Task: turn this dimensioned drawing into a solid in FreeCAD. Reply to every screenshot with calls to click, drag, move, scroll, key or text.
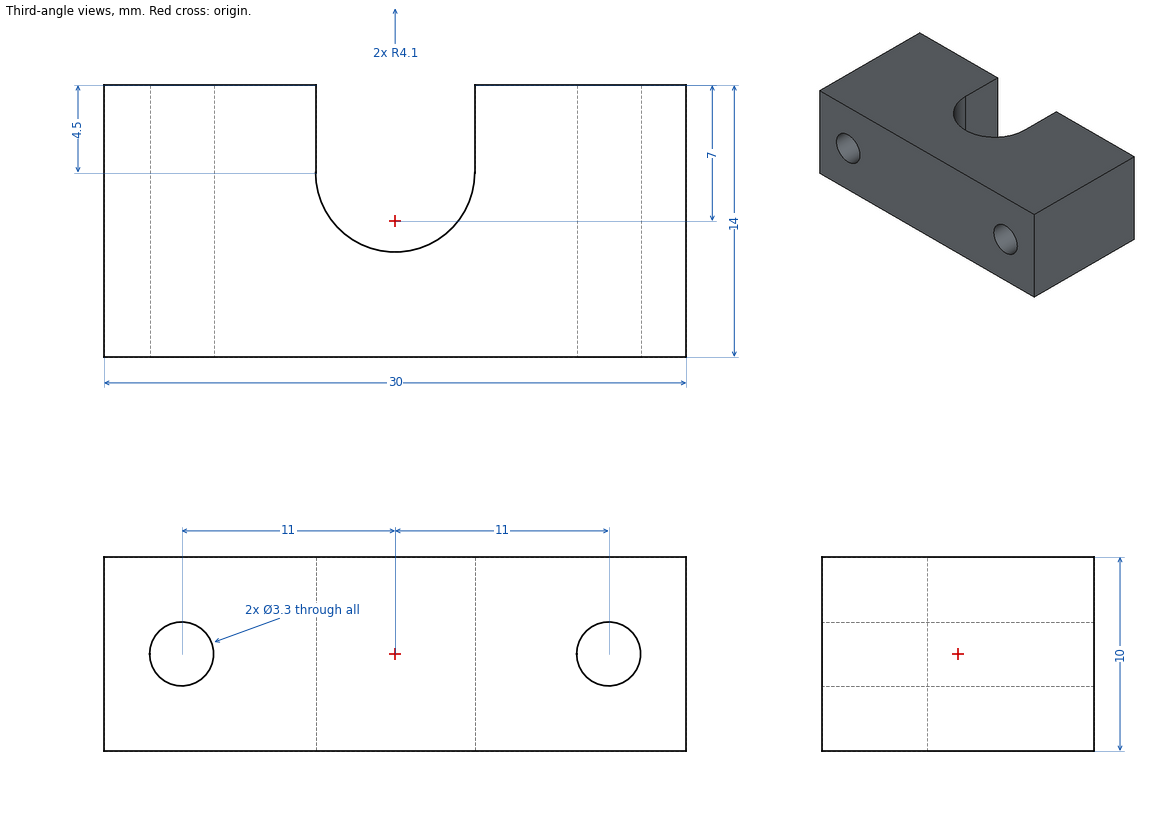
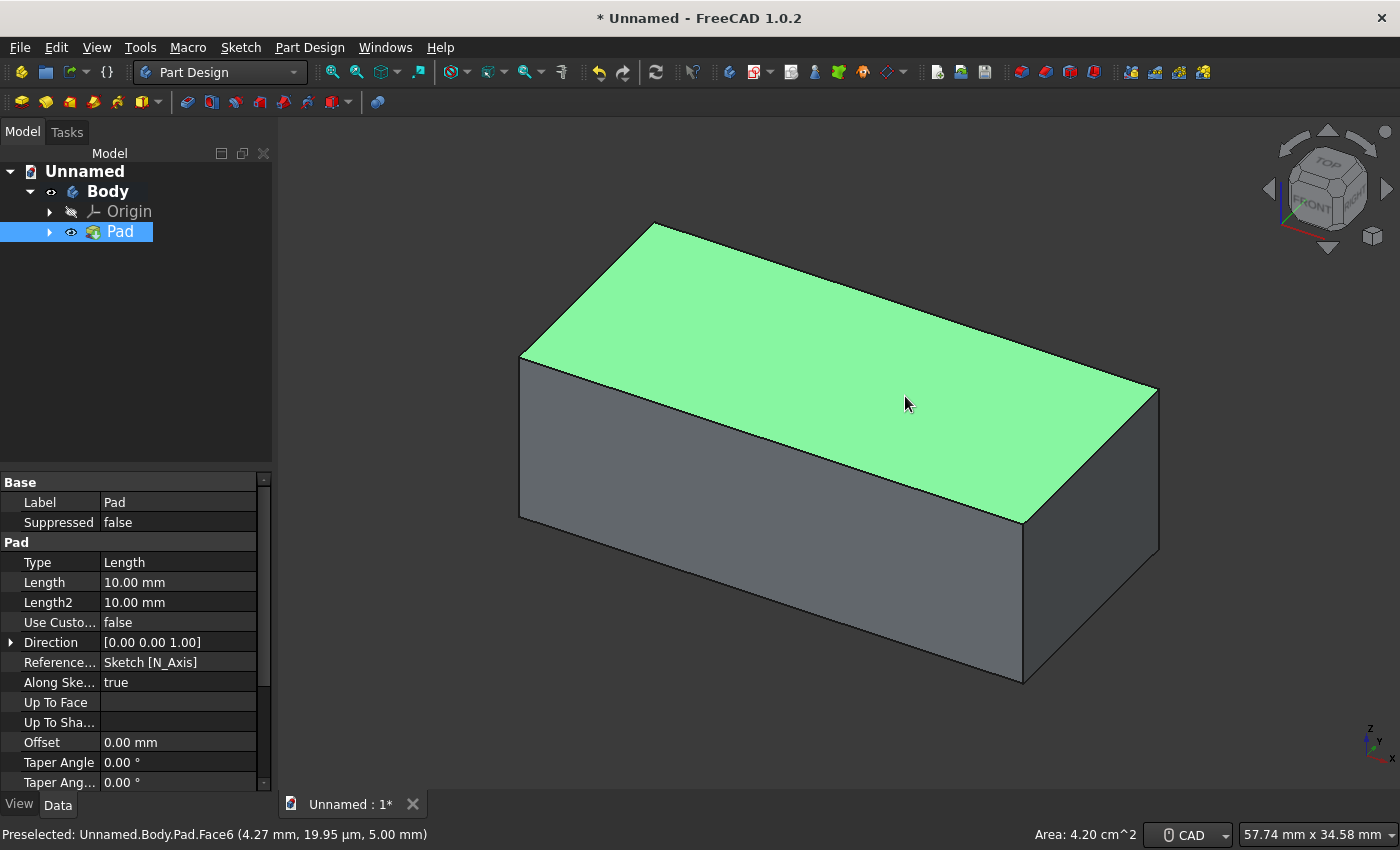
click(754, 72)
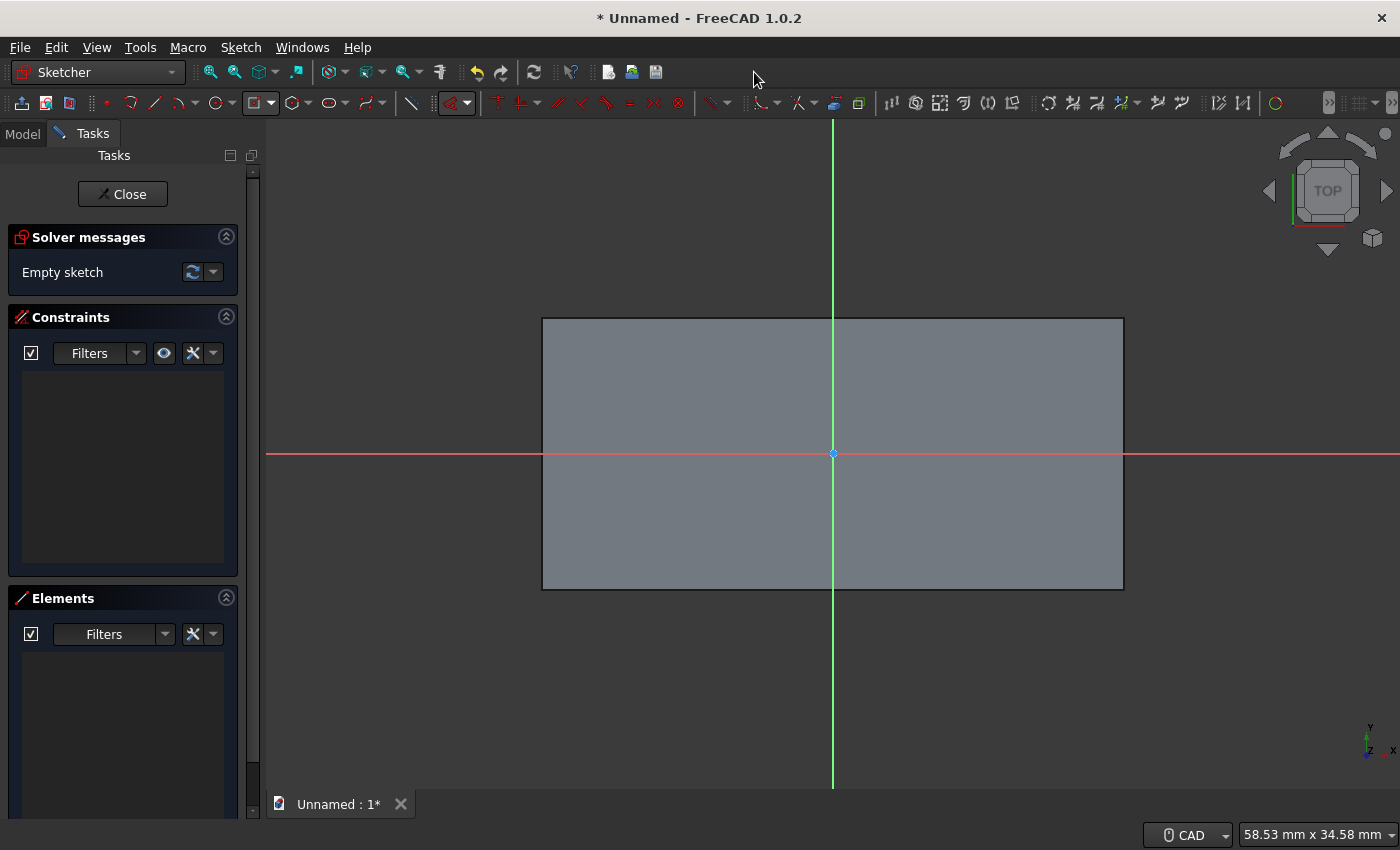
scroll(916, 250, up, 3)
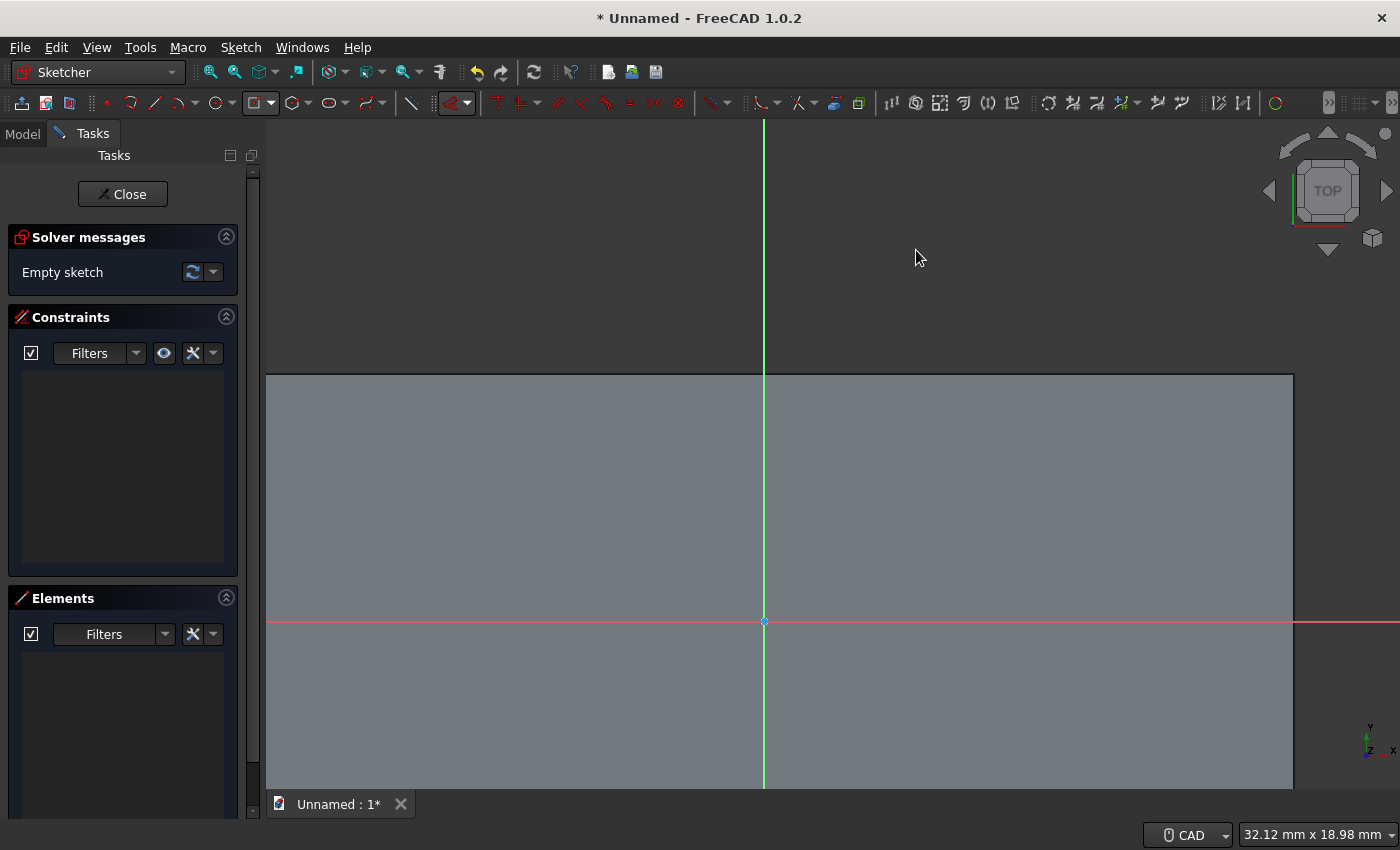
click(330, 104)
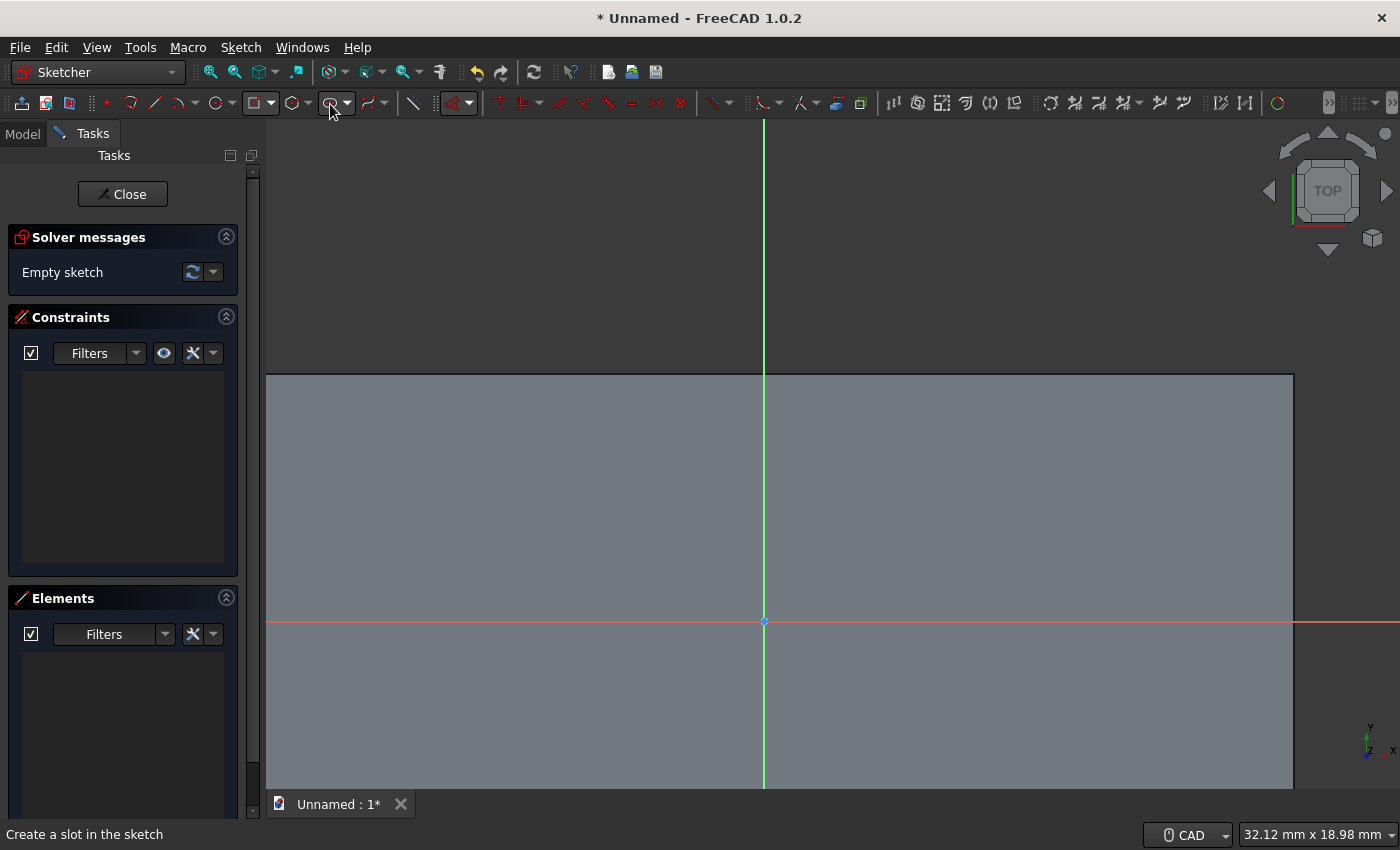
click(764, 533)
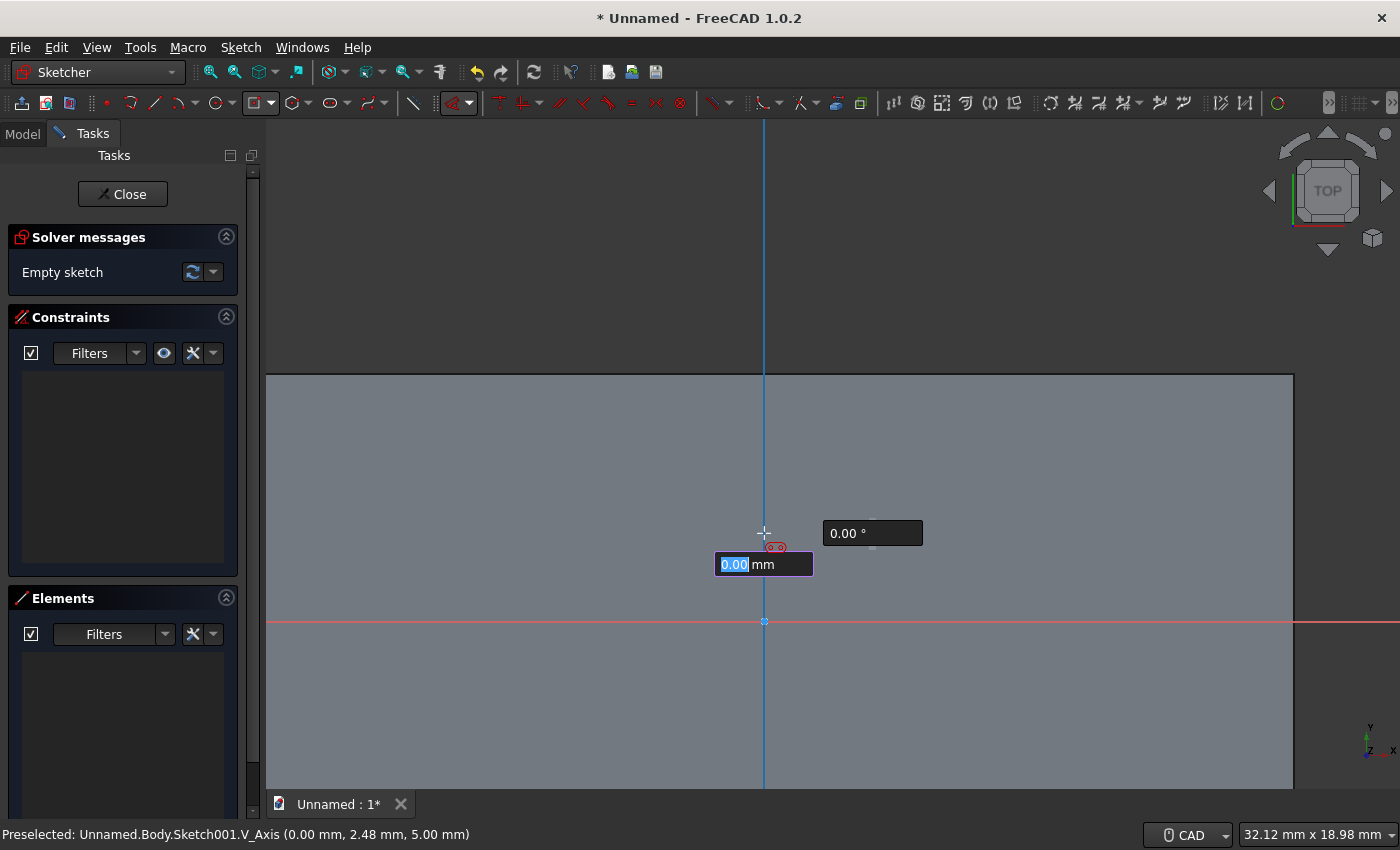
click(773, 374)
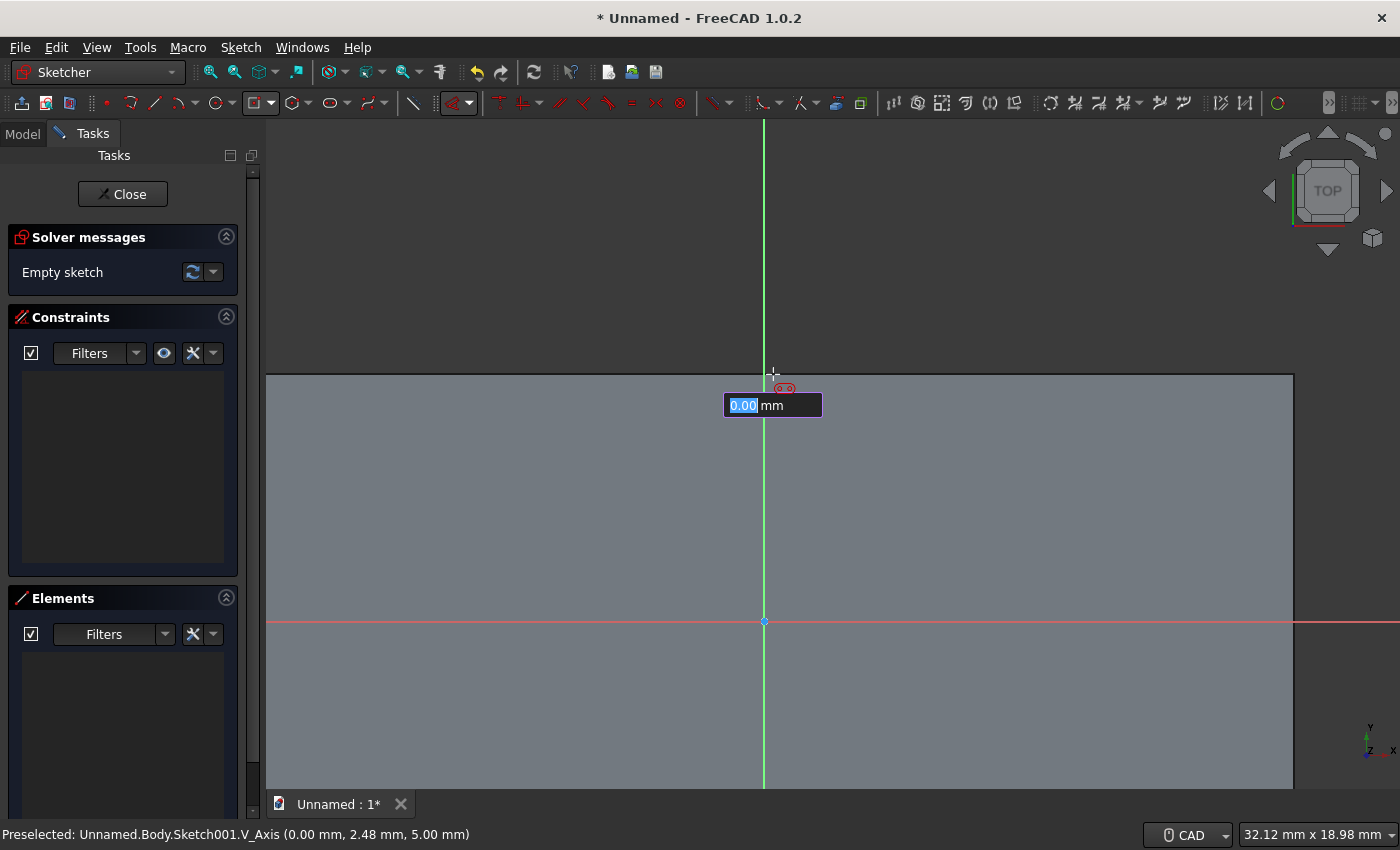
click(909, 454)
key(Escape)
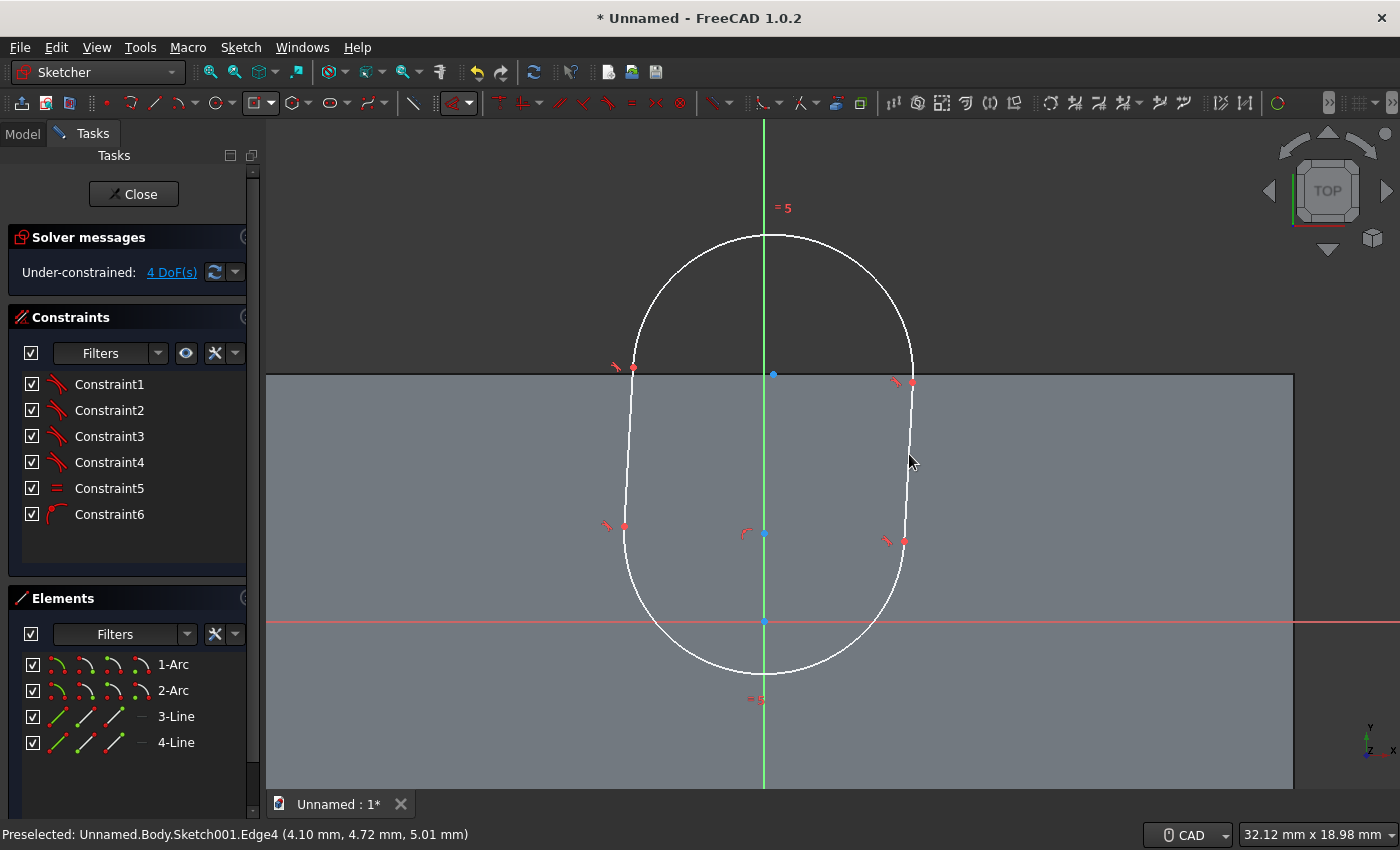
click(627, 479)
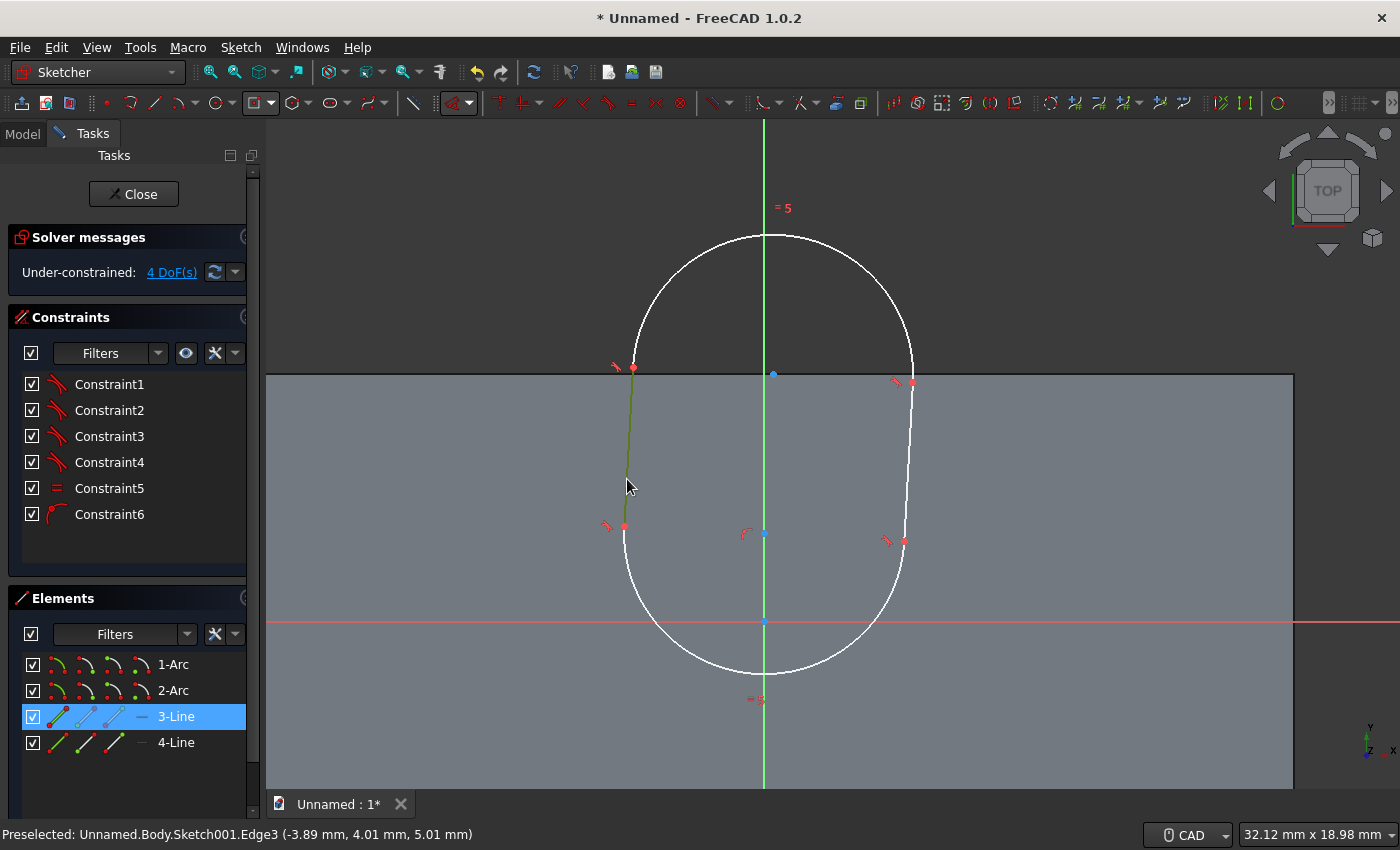
key(v)